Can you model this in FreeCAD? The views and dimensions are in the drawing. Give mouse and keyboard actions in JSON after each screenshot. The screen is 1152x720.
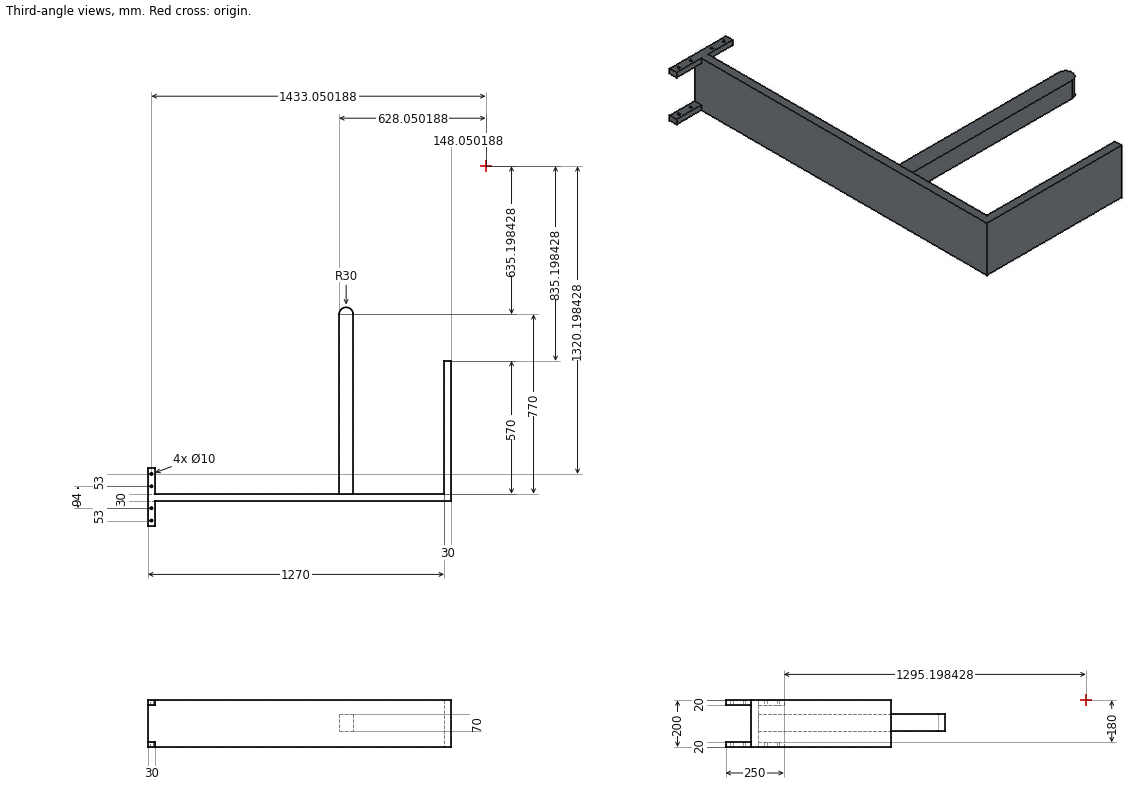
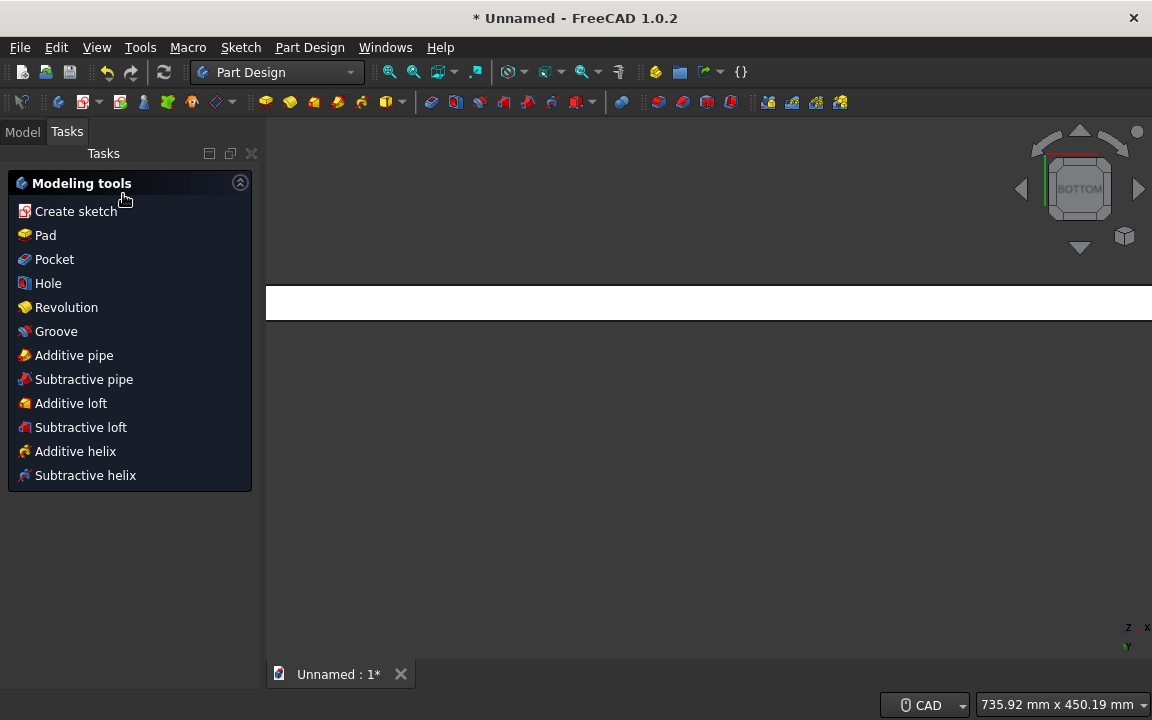
{"action": "left_click", "coordinate": [432, 102]}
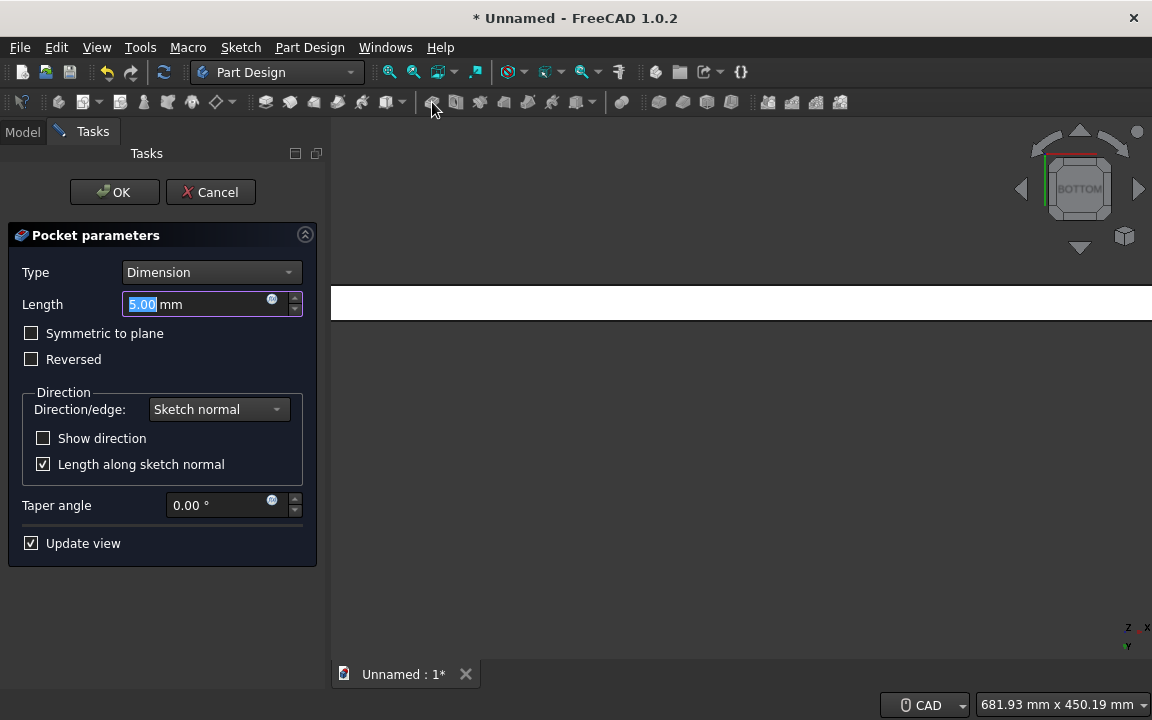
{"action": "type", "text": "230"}
{"action": "key", "text": "Tab"}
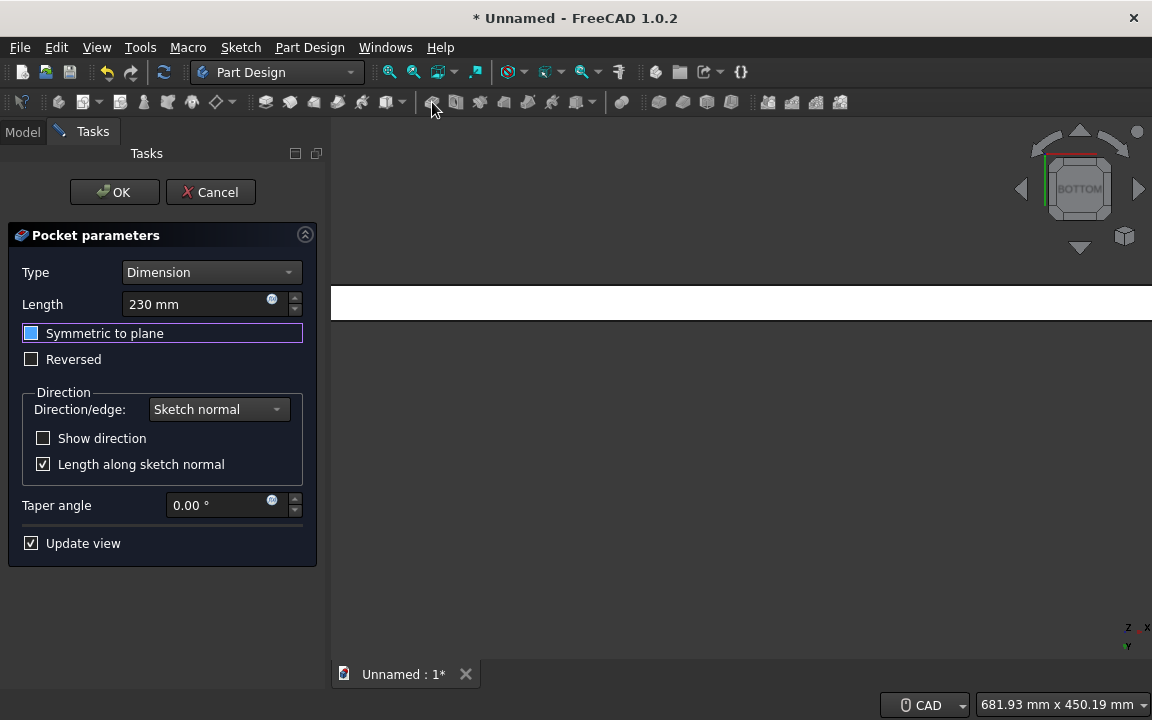
{"action": "left_click", "coordinate": [115, 192]}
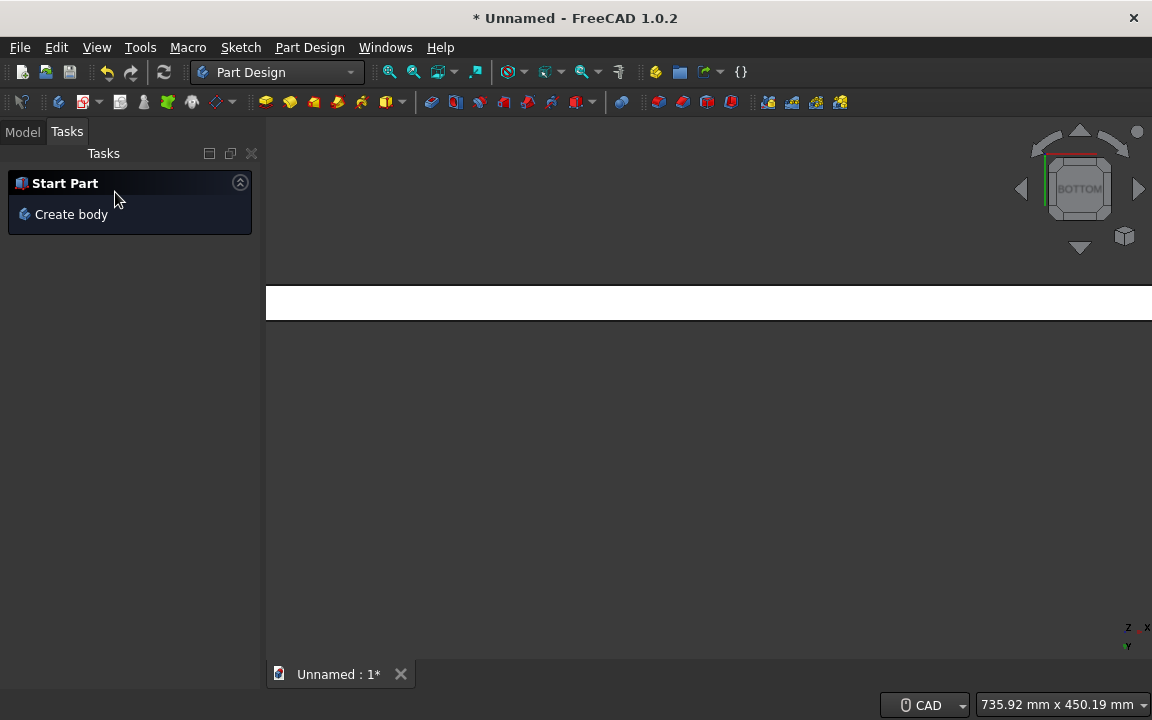
{"action": "left_click", "coordinate": [390, 72]}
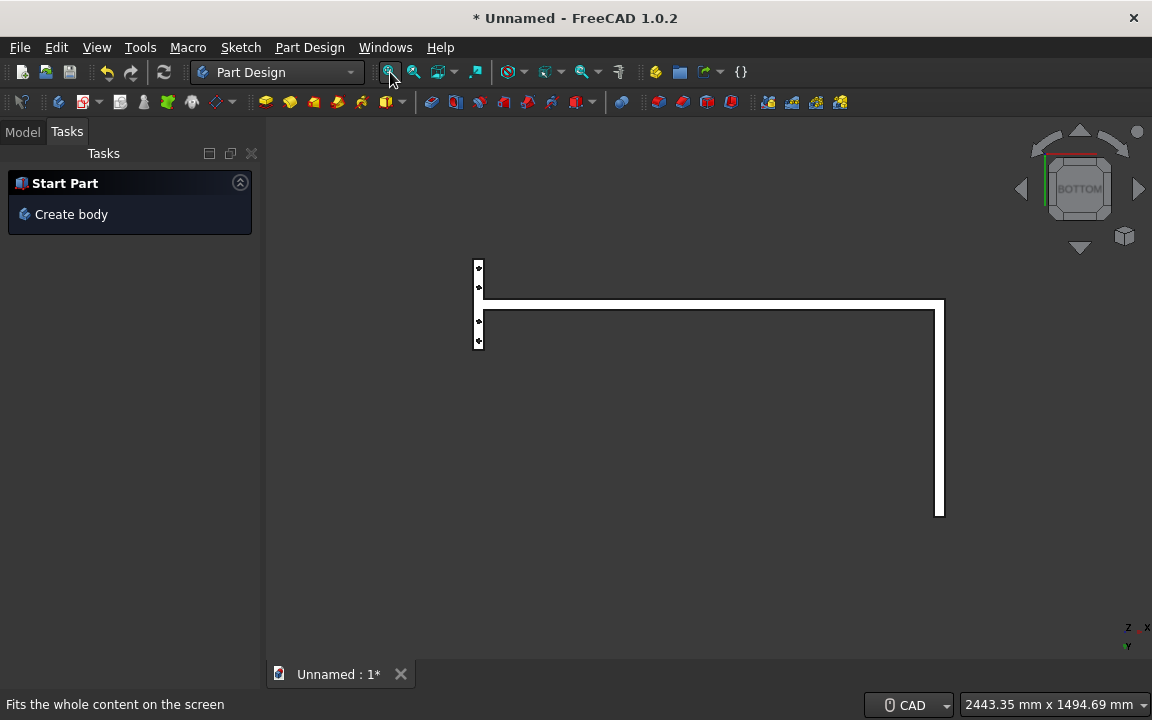
{"action": "left_click", "coordinate": [23, 131]}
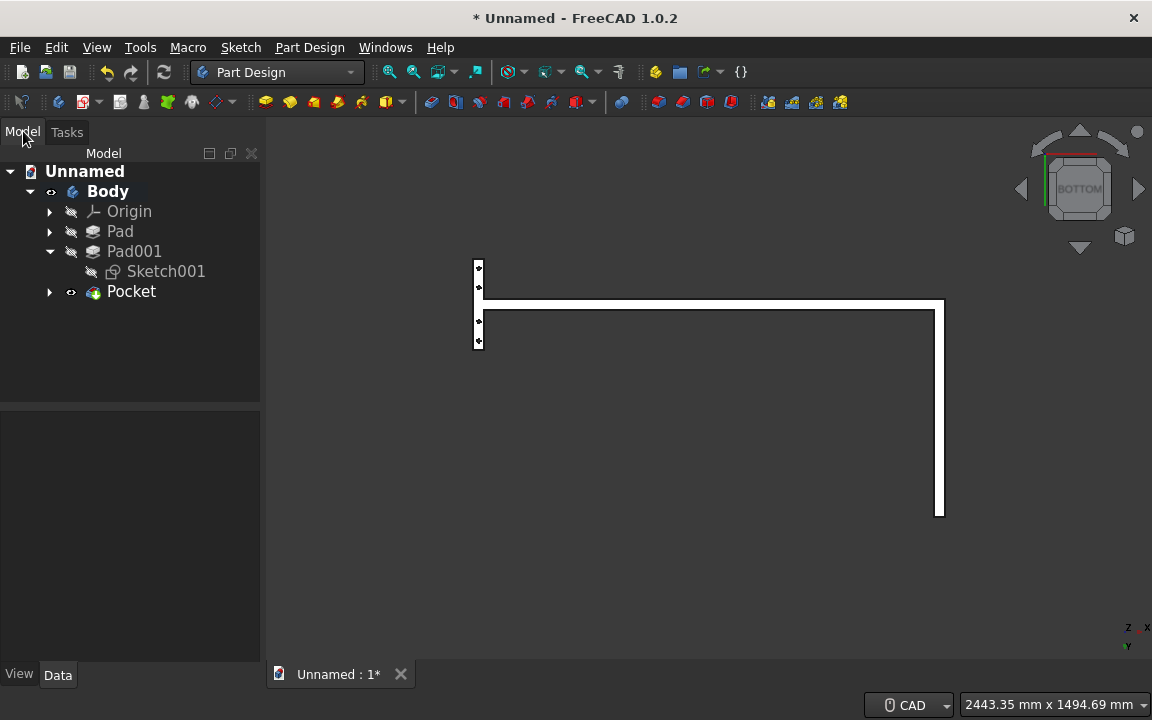
{"action": "left_click", "coordinate": [50, 212]}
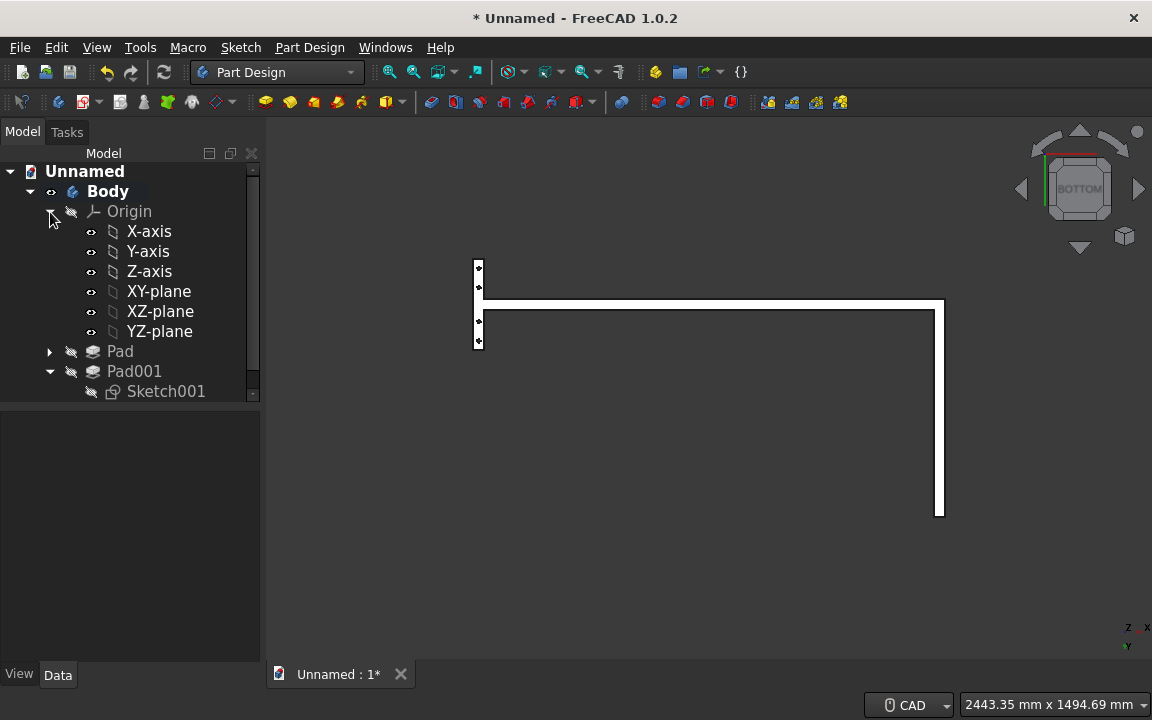
{"action": "left_click", "coordinate": [136, 292]}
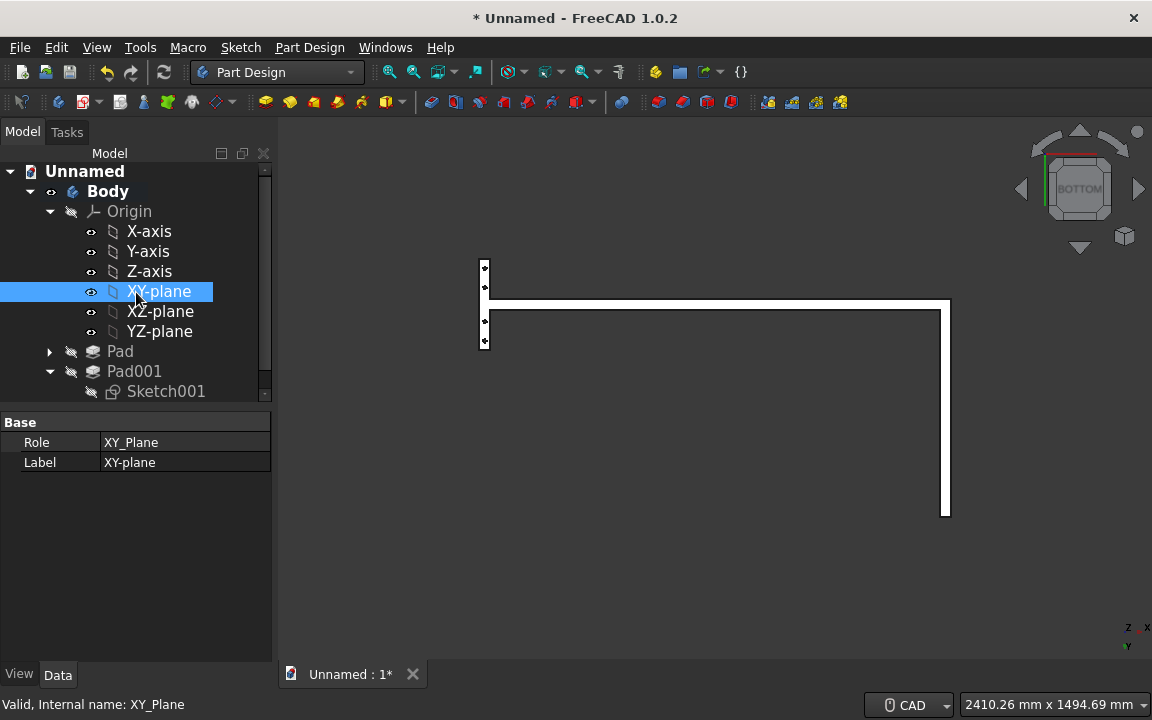
{"action": "left_click", "coordinate": [216, 102]}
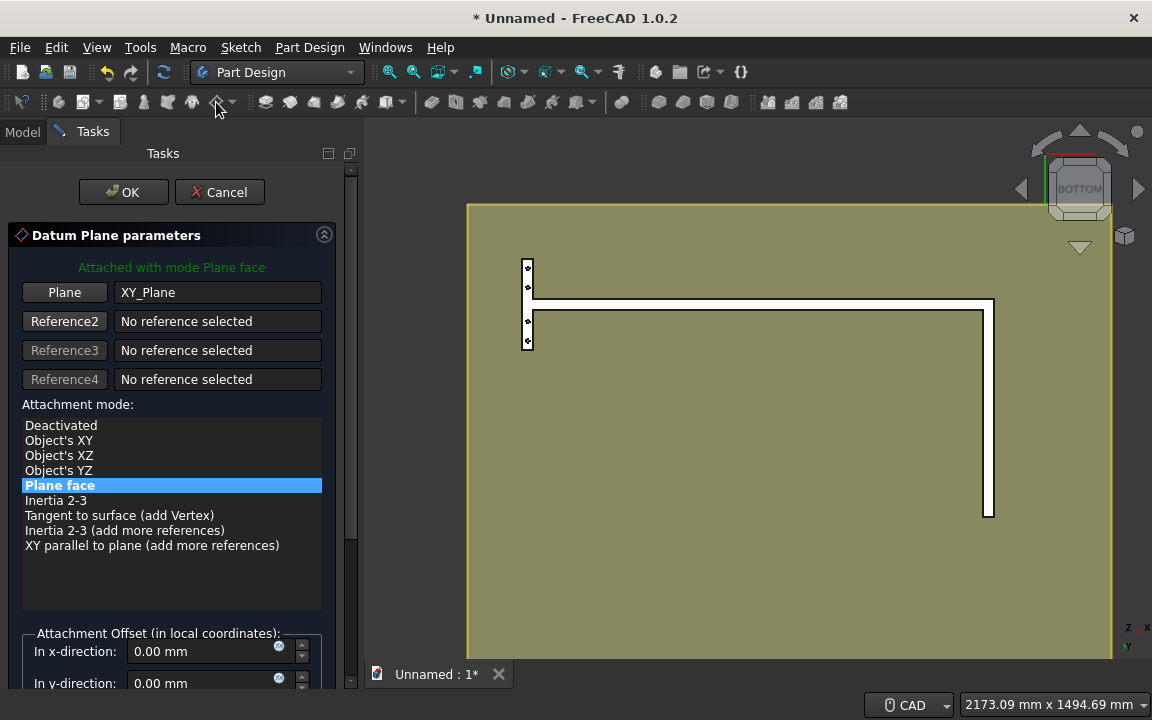
{"action": "scroll", "coordinate": [351, 426], "scroll_direction": "down", "scroll_amount": 2}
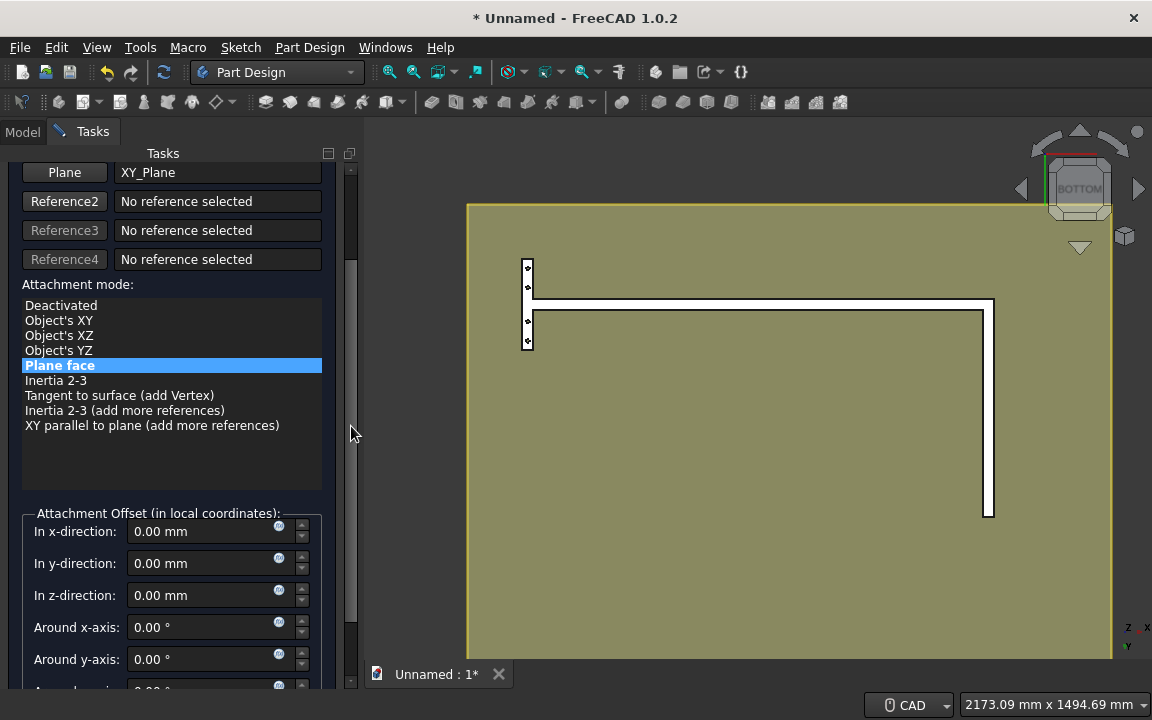
{"action": "triple_click", "coordinate": [210, 595]}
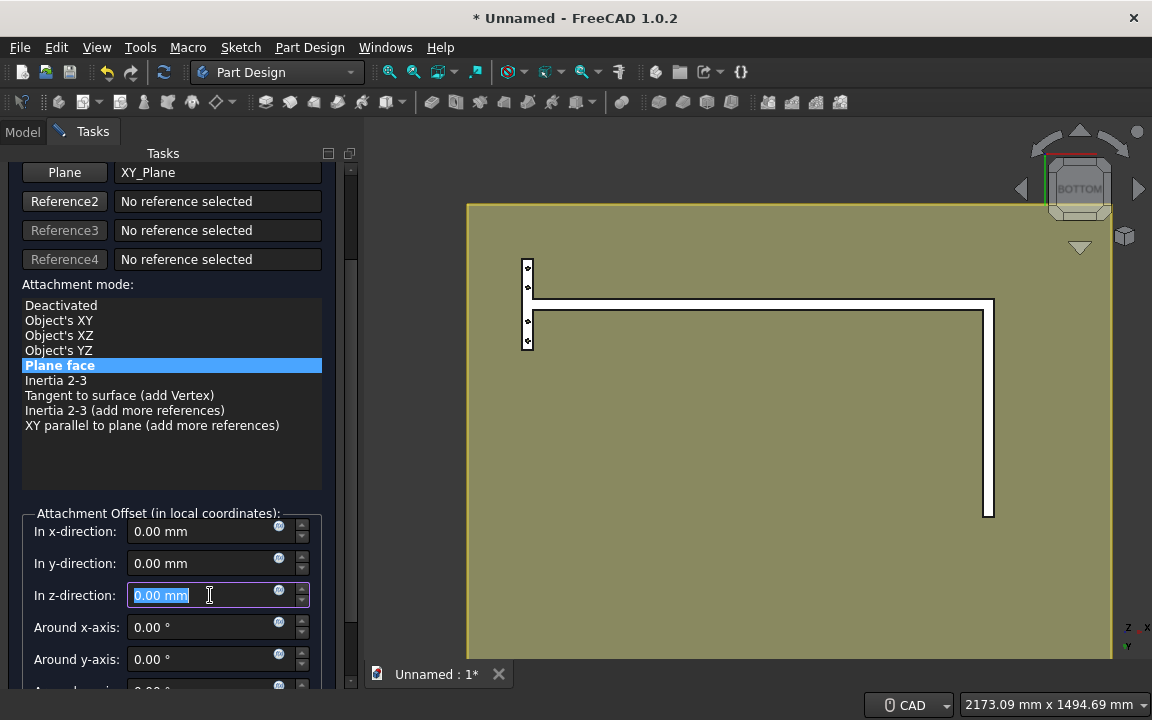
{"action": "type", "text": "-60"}
{"action": "key", "text": "Tab"}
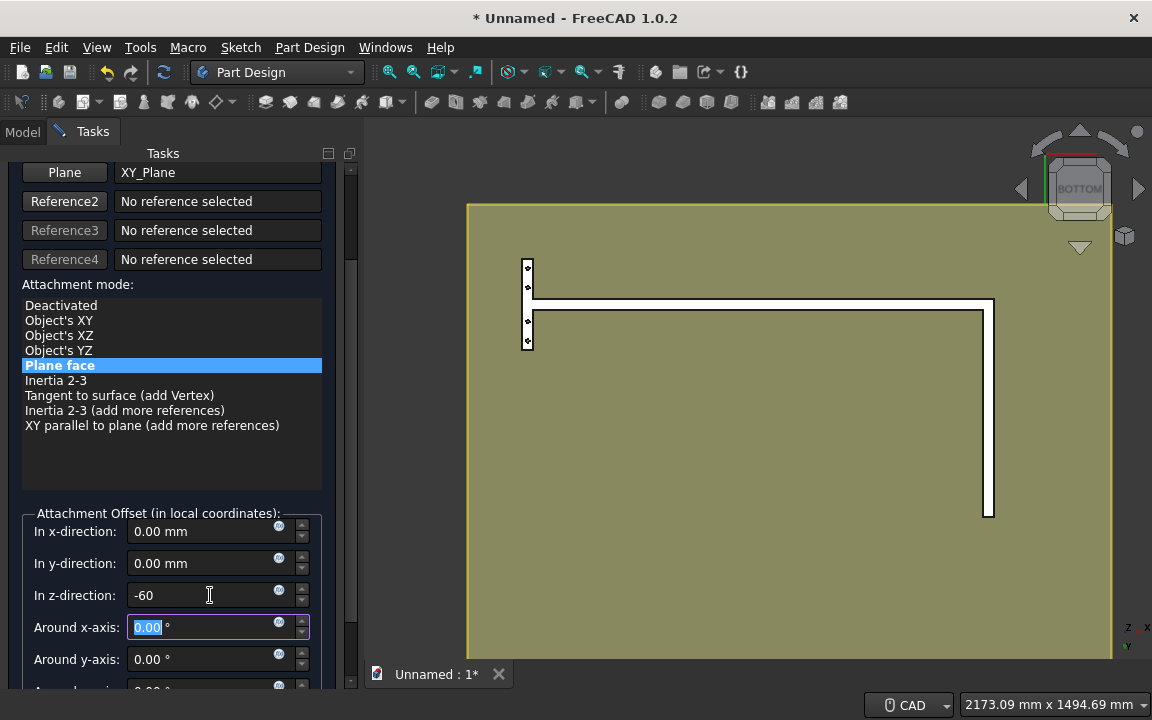
{"action": "scroll", "coordinate": [351, 426], "scroll_direction": "up", "scroll_amount": 3}